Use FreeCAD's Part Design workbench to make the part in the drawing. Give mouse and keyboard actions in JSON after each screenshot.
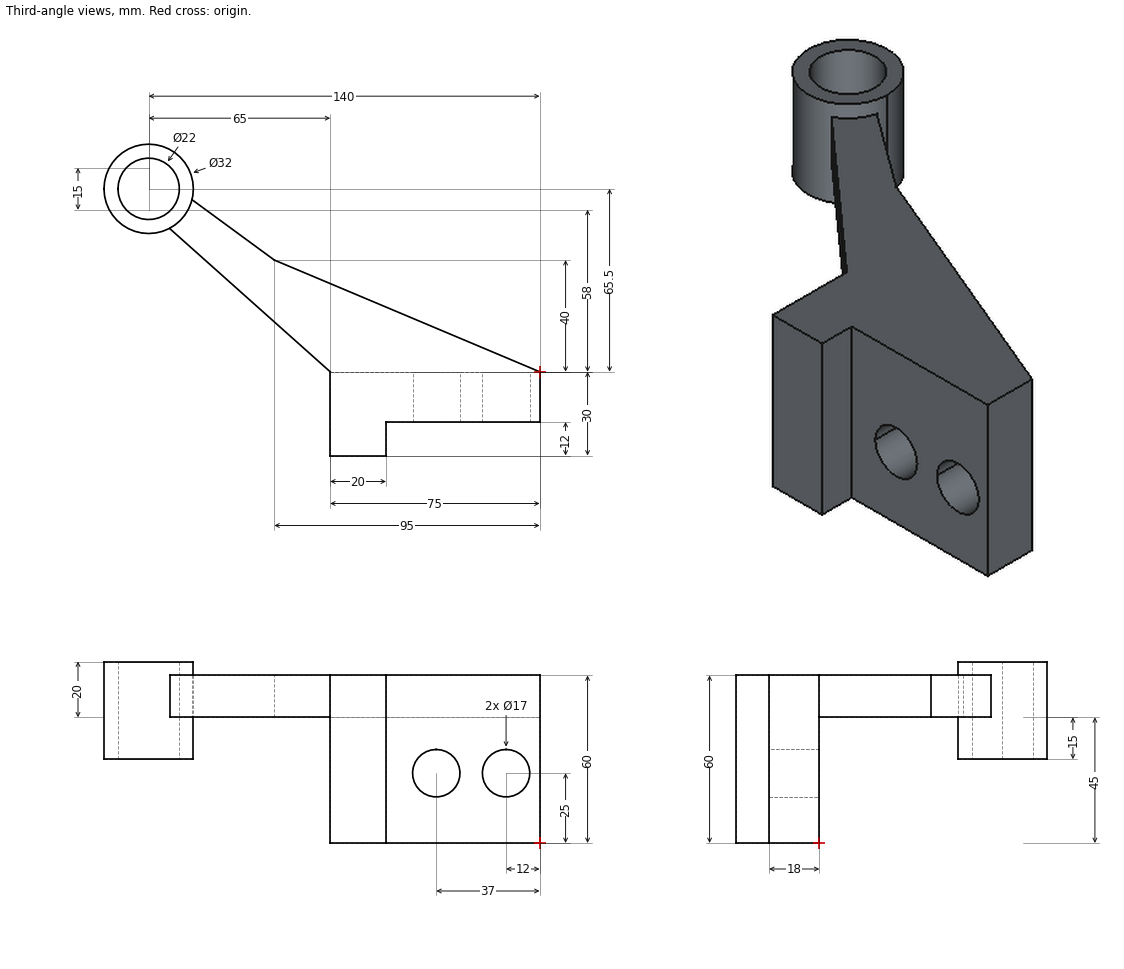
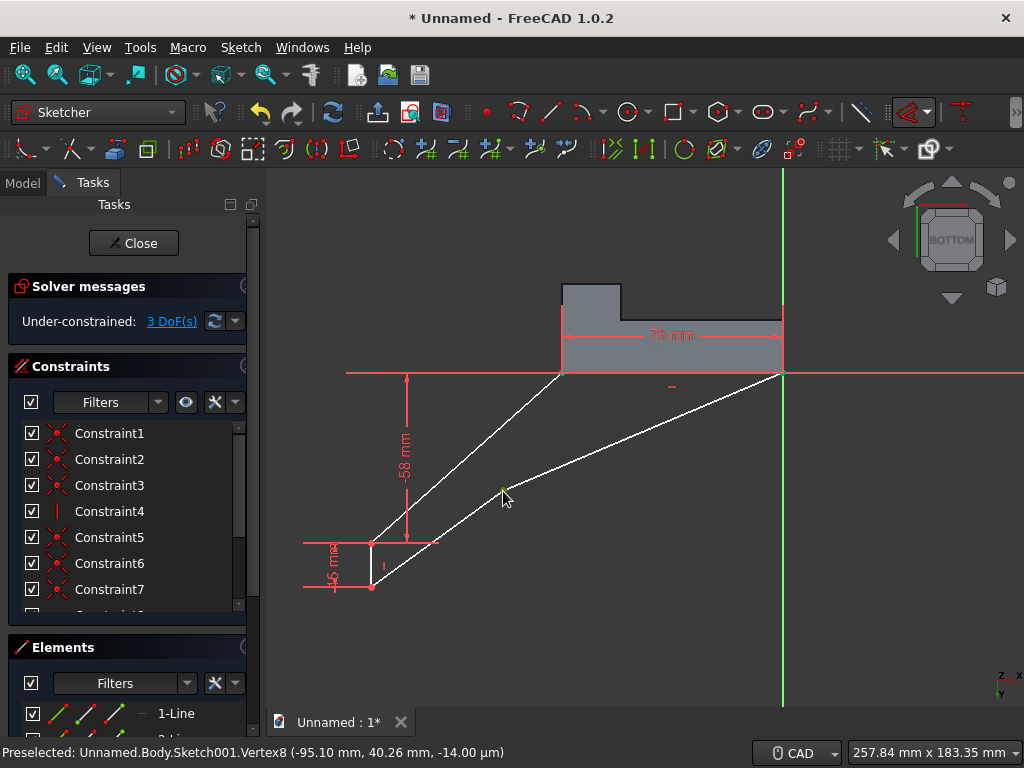
{"action": "left_click", "coordinate": [930, 112]}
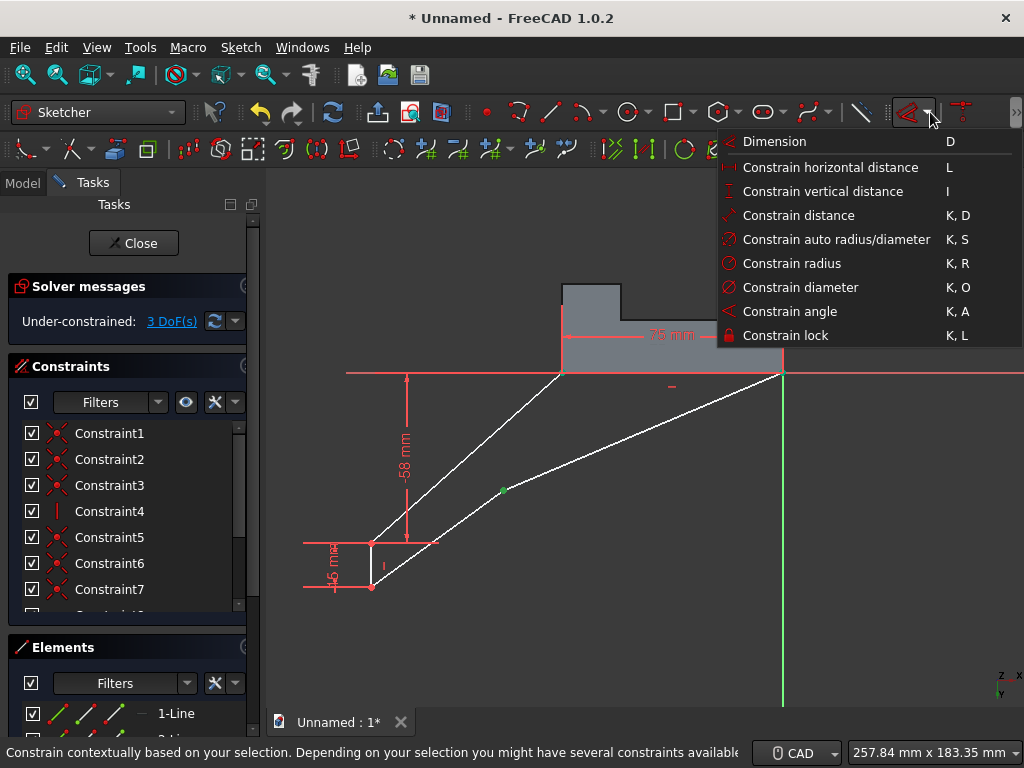
{"action": "left_click", "coordinate": [870, 167]}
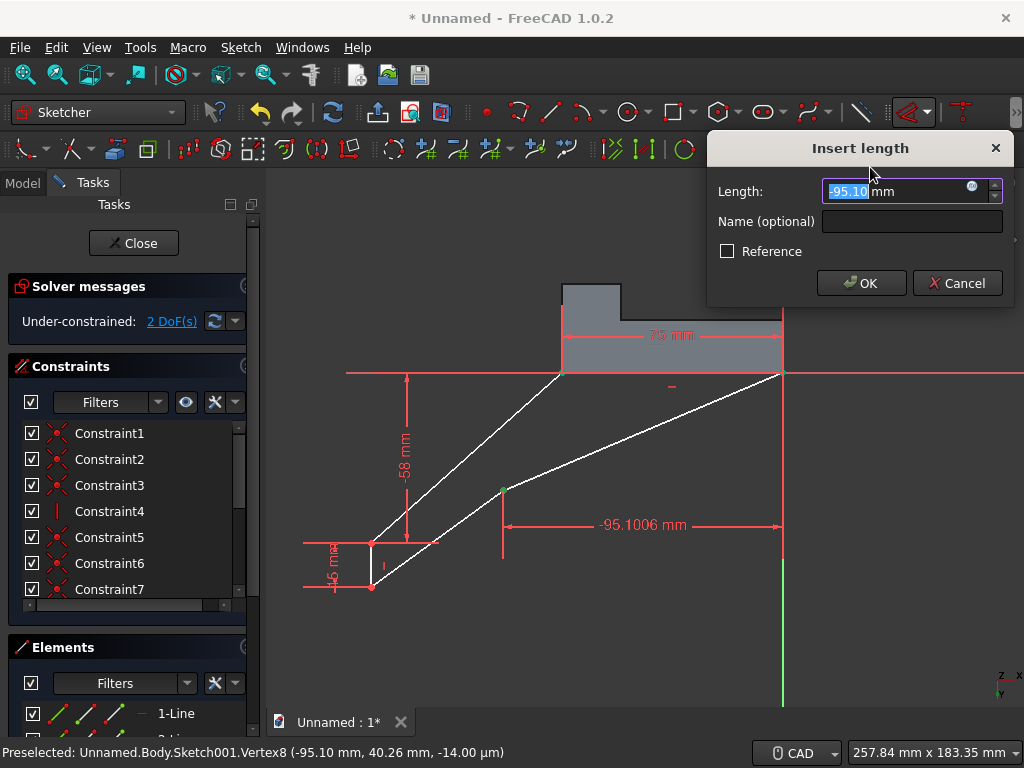
{"action": "type", "text": "-95"}
{"action": "key", "text": "Return"}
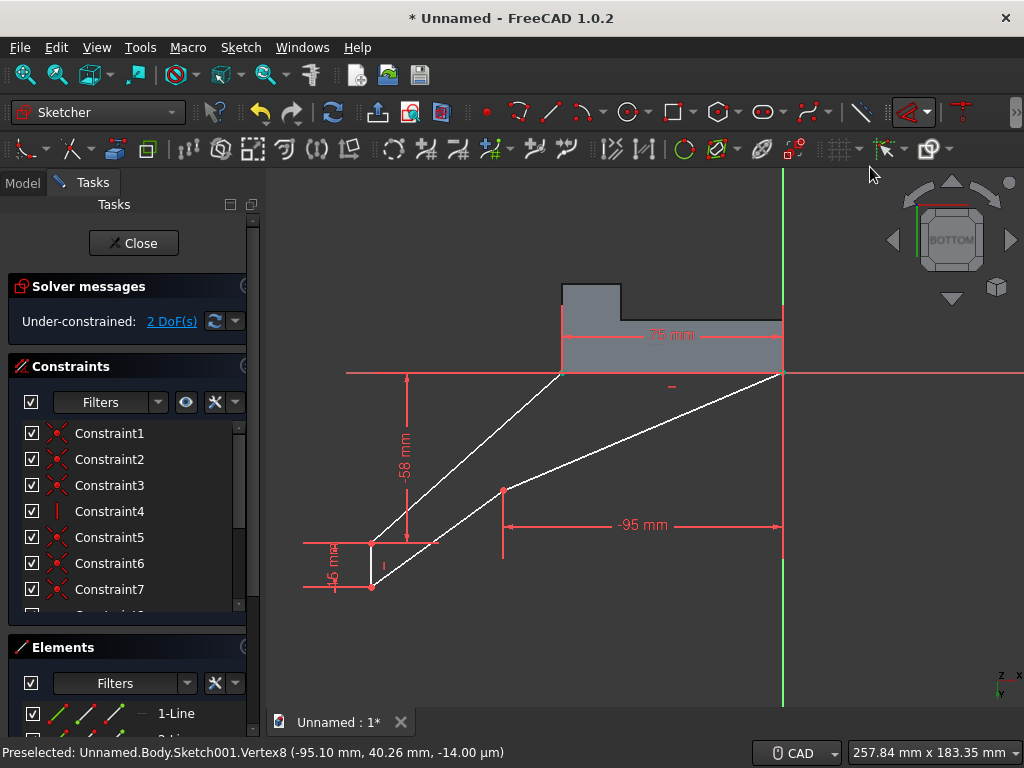
{"action": "left_click", "coordinate": [503, 491]}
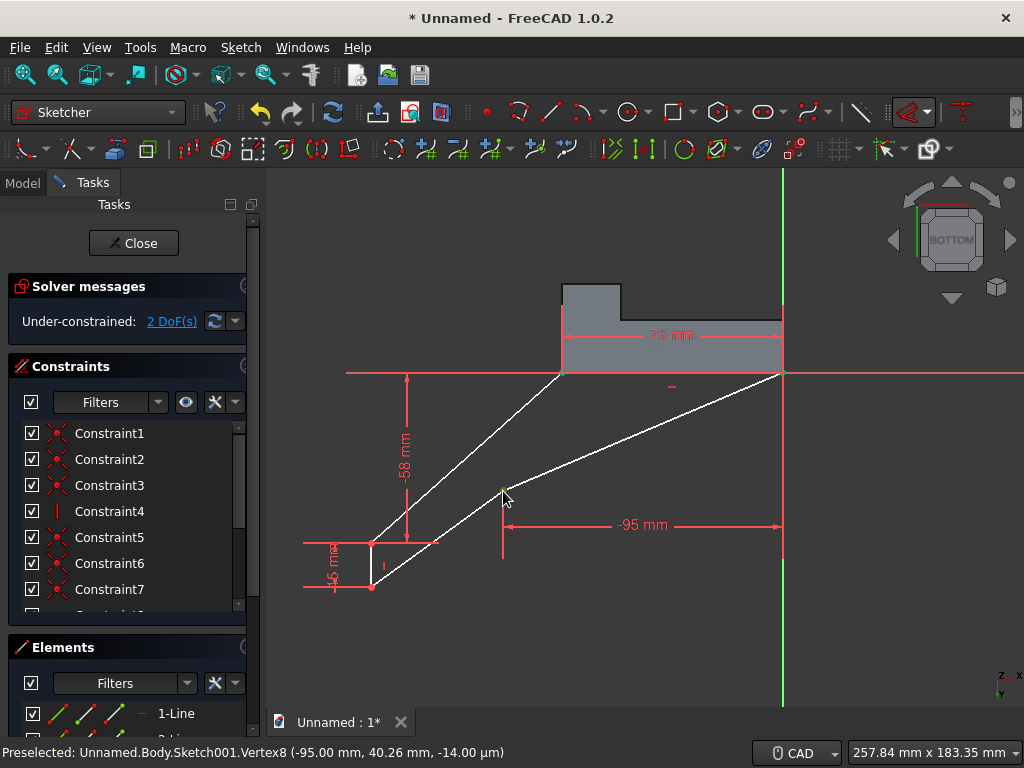
{"action": "left_click", "coordinate": [930, 112]}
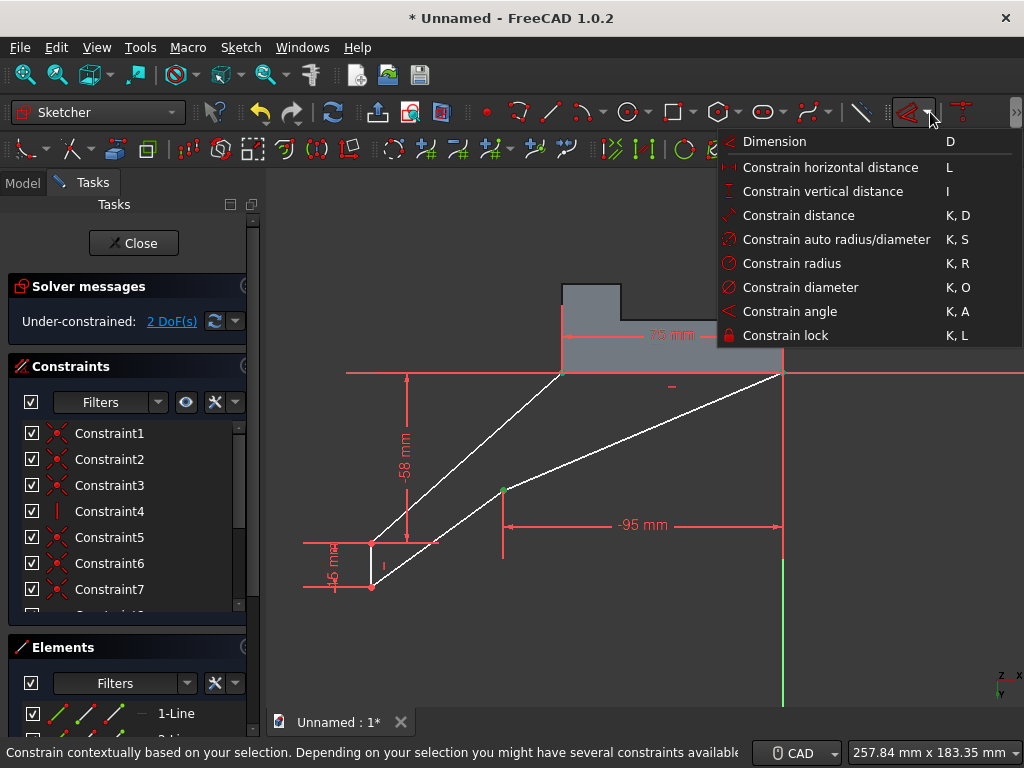
{"action": "left_click", "coordinate": [870, 191]}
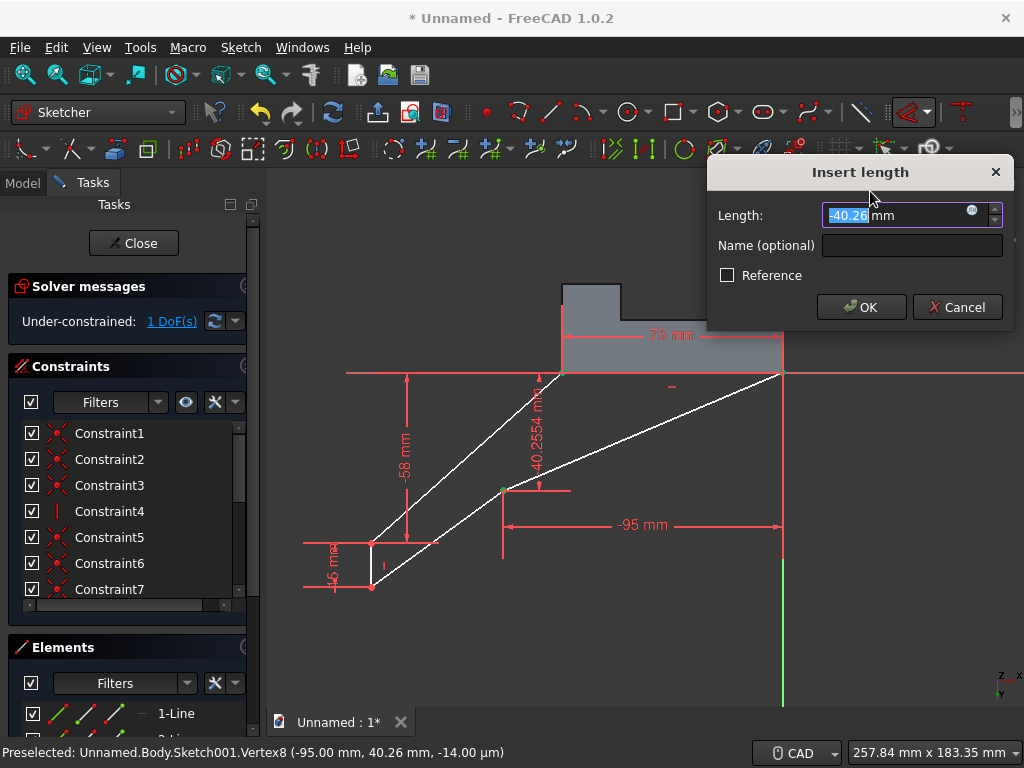
{"action": "type", "text": "-40"}
{"action": "key", "text": "Return"}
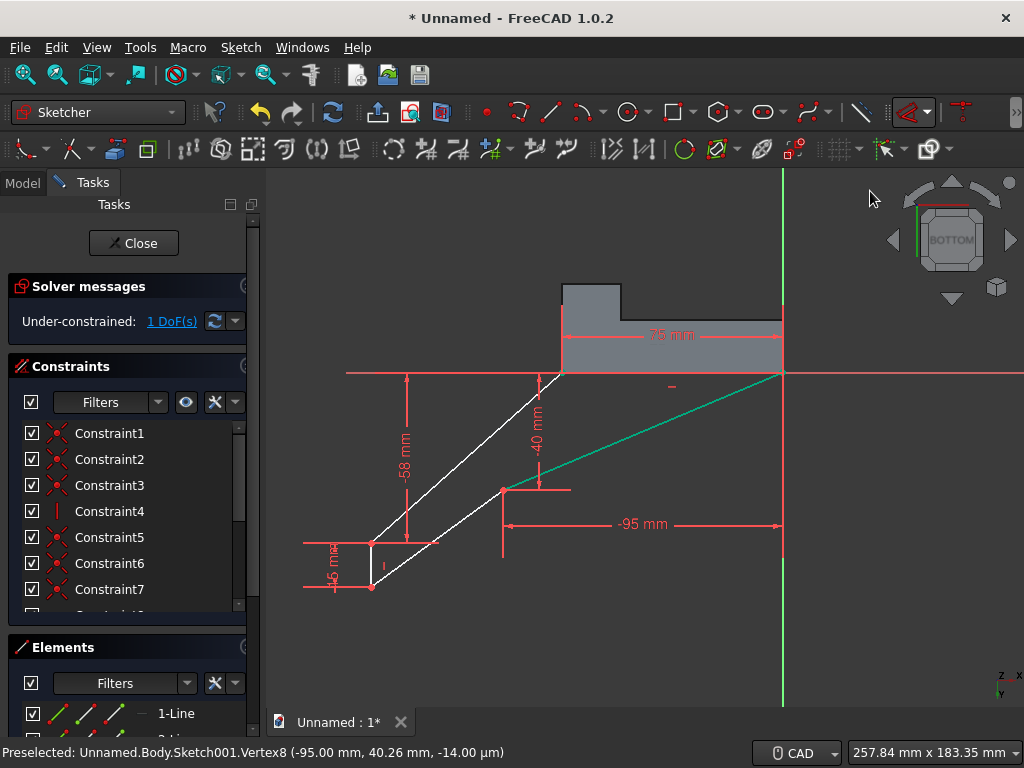
{"action": "left_click", "coordinate": [505, 424]}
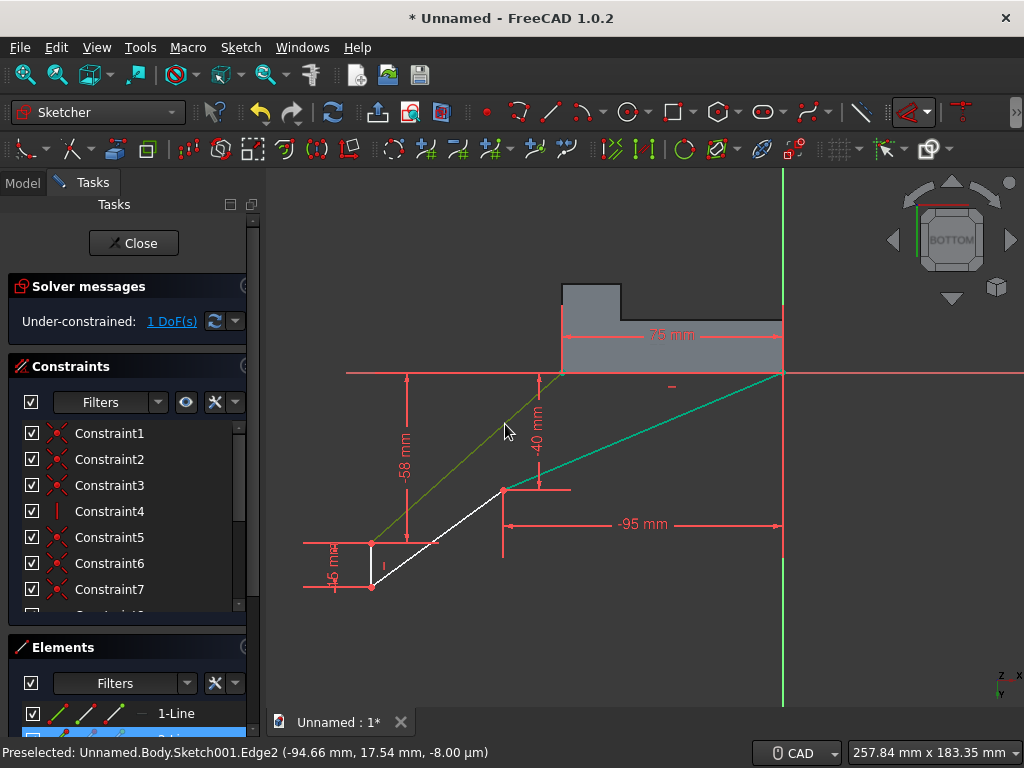
{"action": "left_click", "coordinate": [930, 112]}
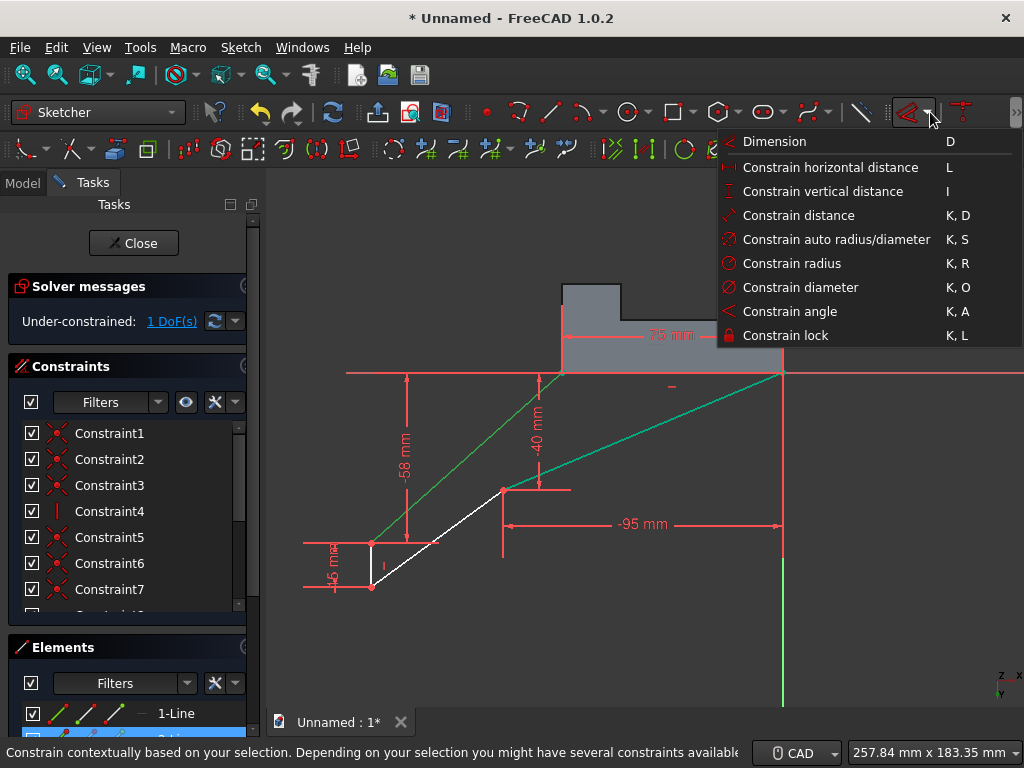
{"action": "left_click", "coordinate": [870, 167]}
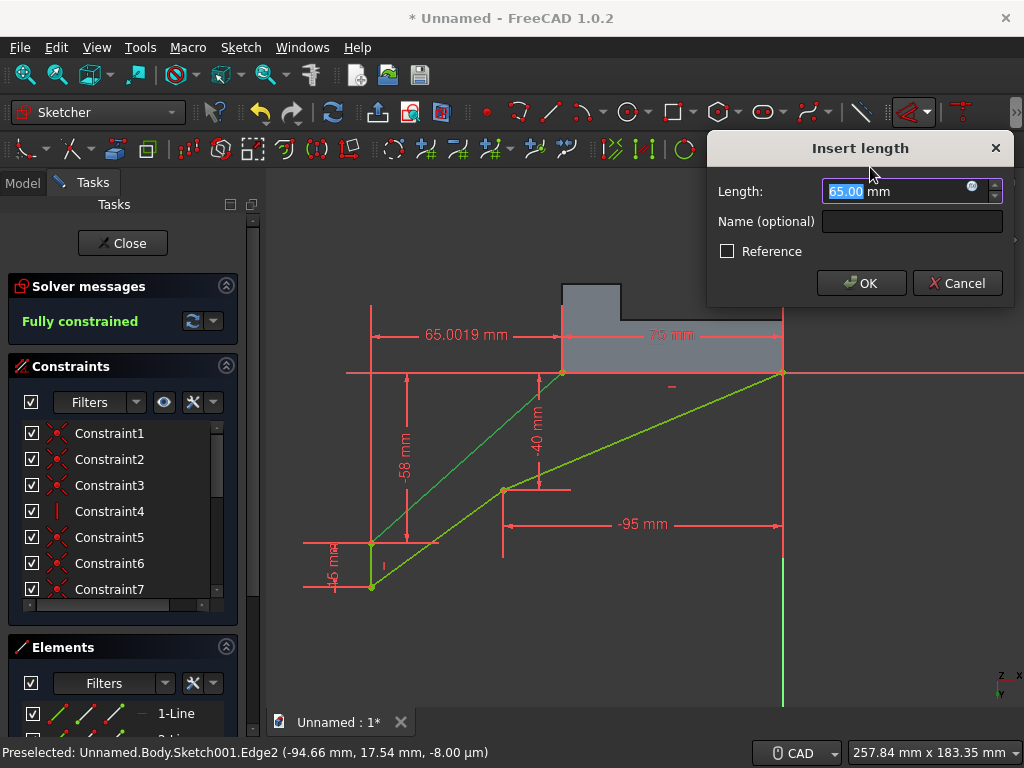
{"action": "type", "text": "65"}
{"action": "key", "text": "Return"}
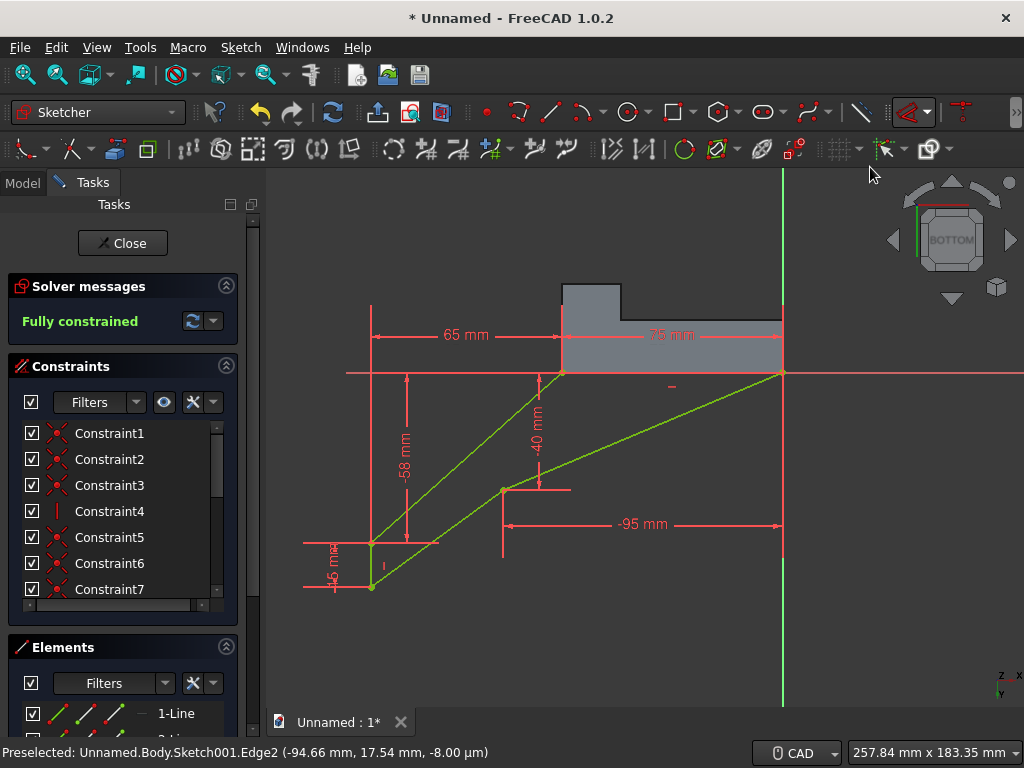
{"action": "left_click", "coordinate": [123, 243]}